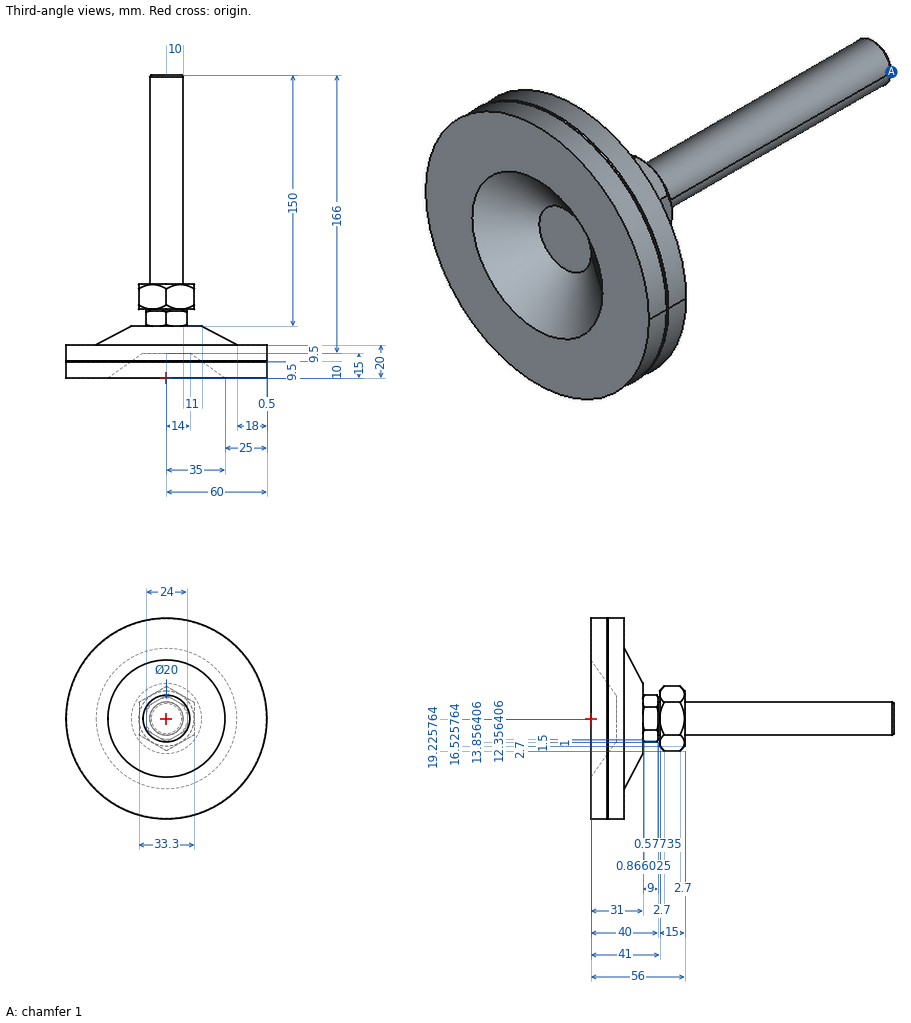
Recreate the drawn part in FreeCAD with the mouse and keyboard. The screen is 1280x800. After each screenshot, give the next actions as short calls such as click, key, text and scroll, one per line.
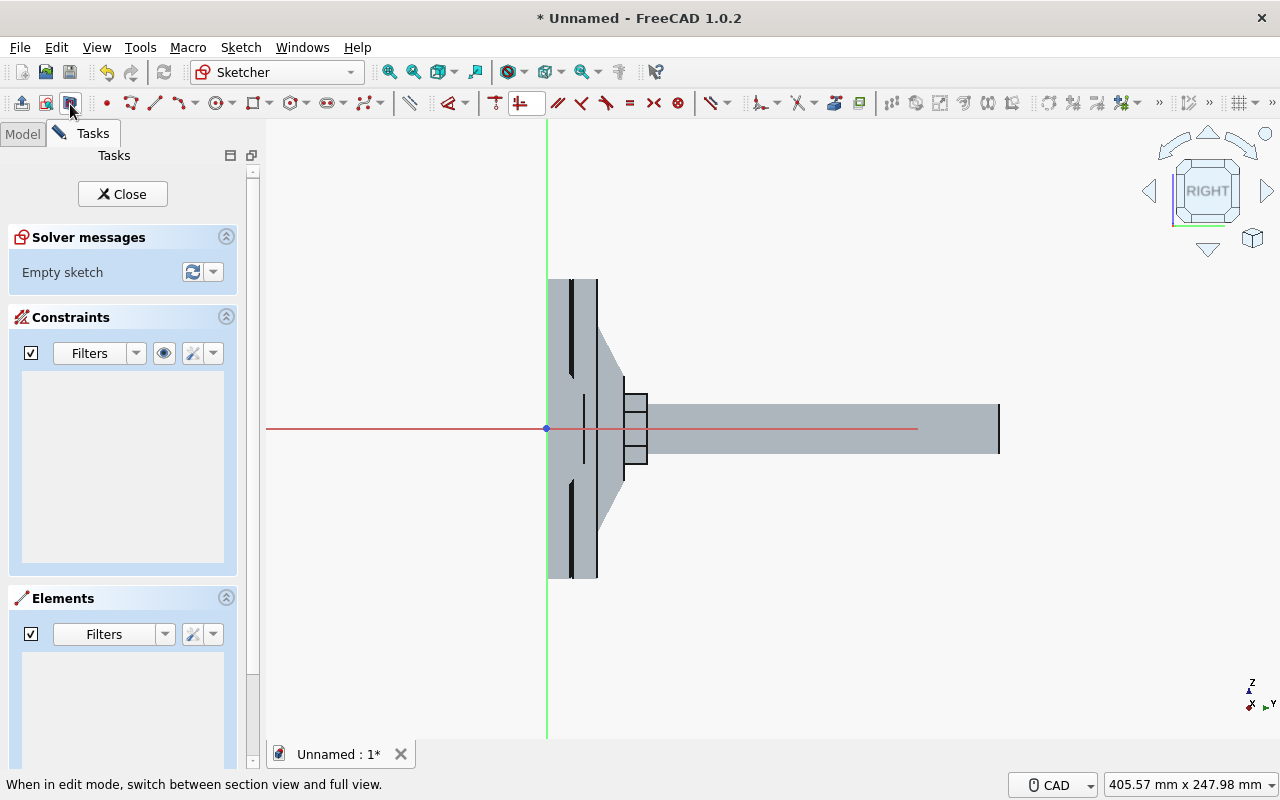
scroll(632, 463, up, 15)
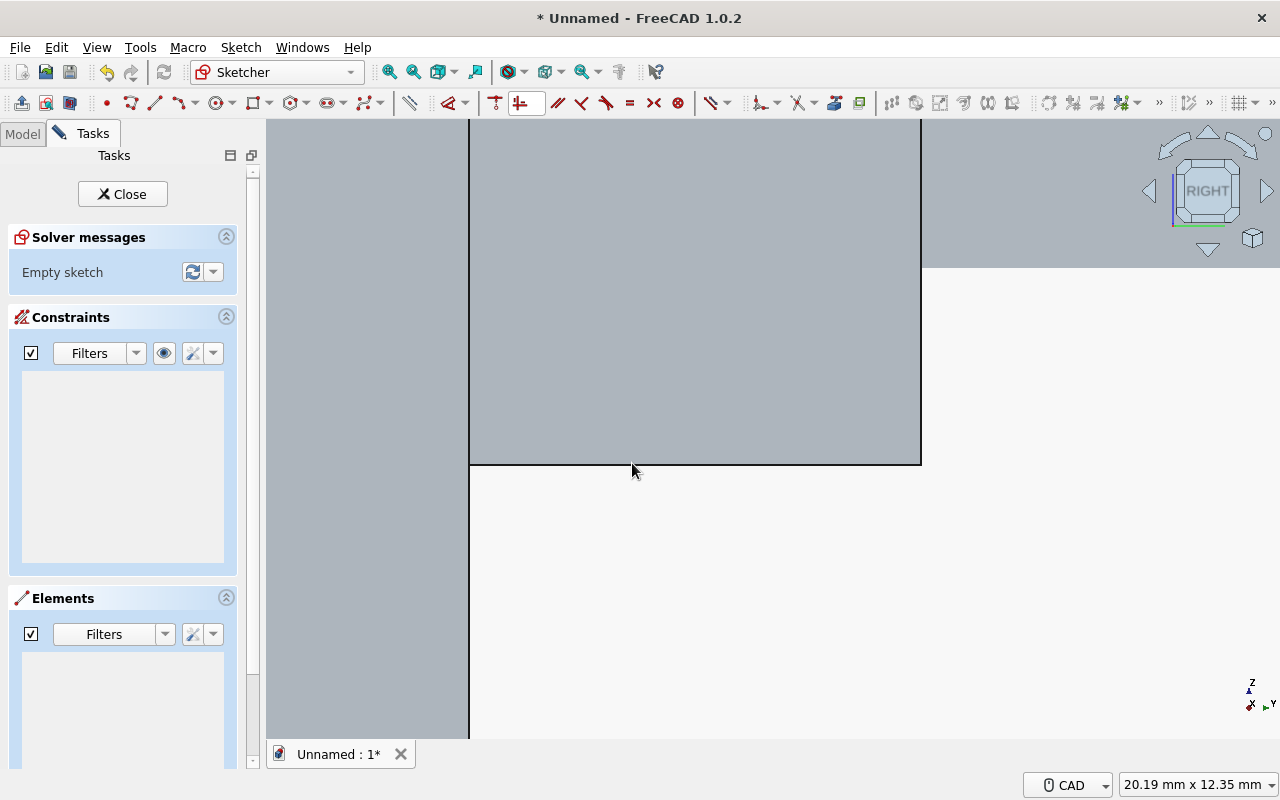
click(132, 104)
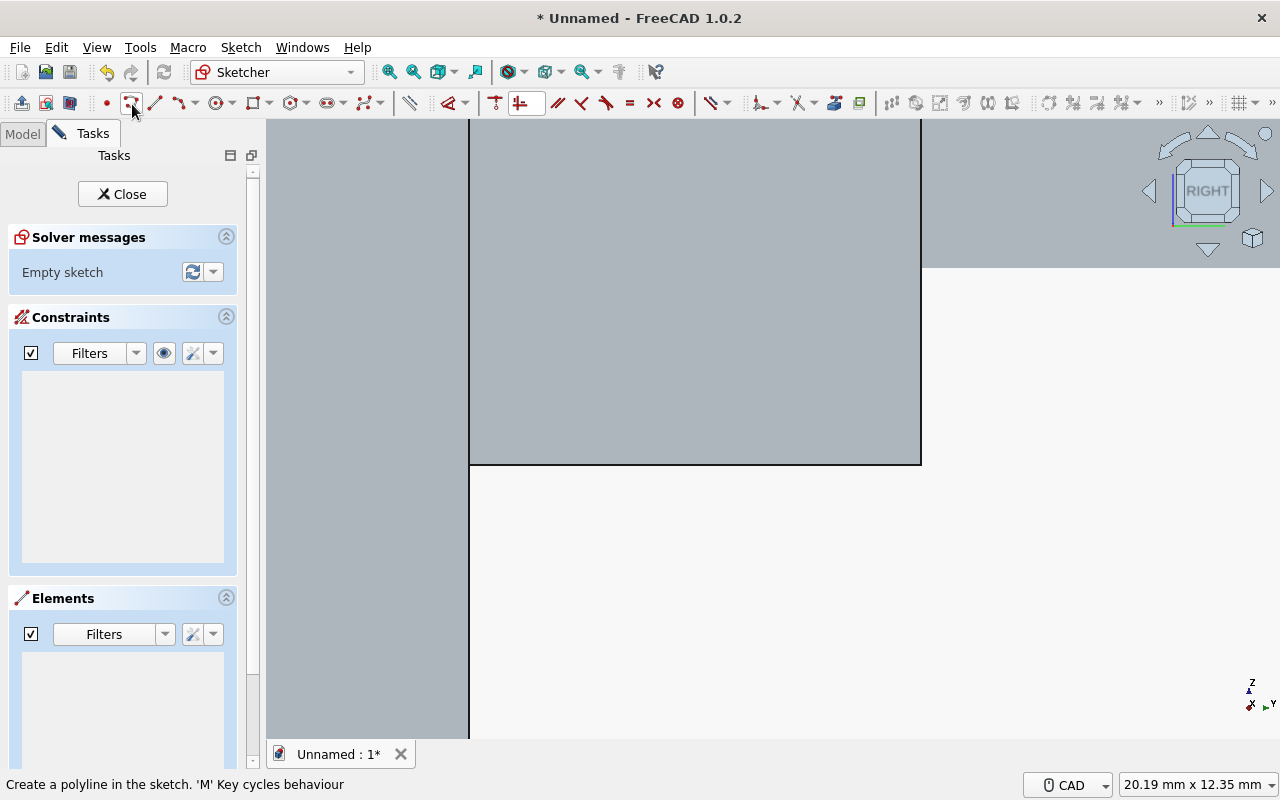
click(469, 390)
click(469, 465)
click(513, 465)
click(469, 391)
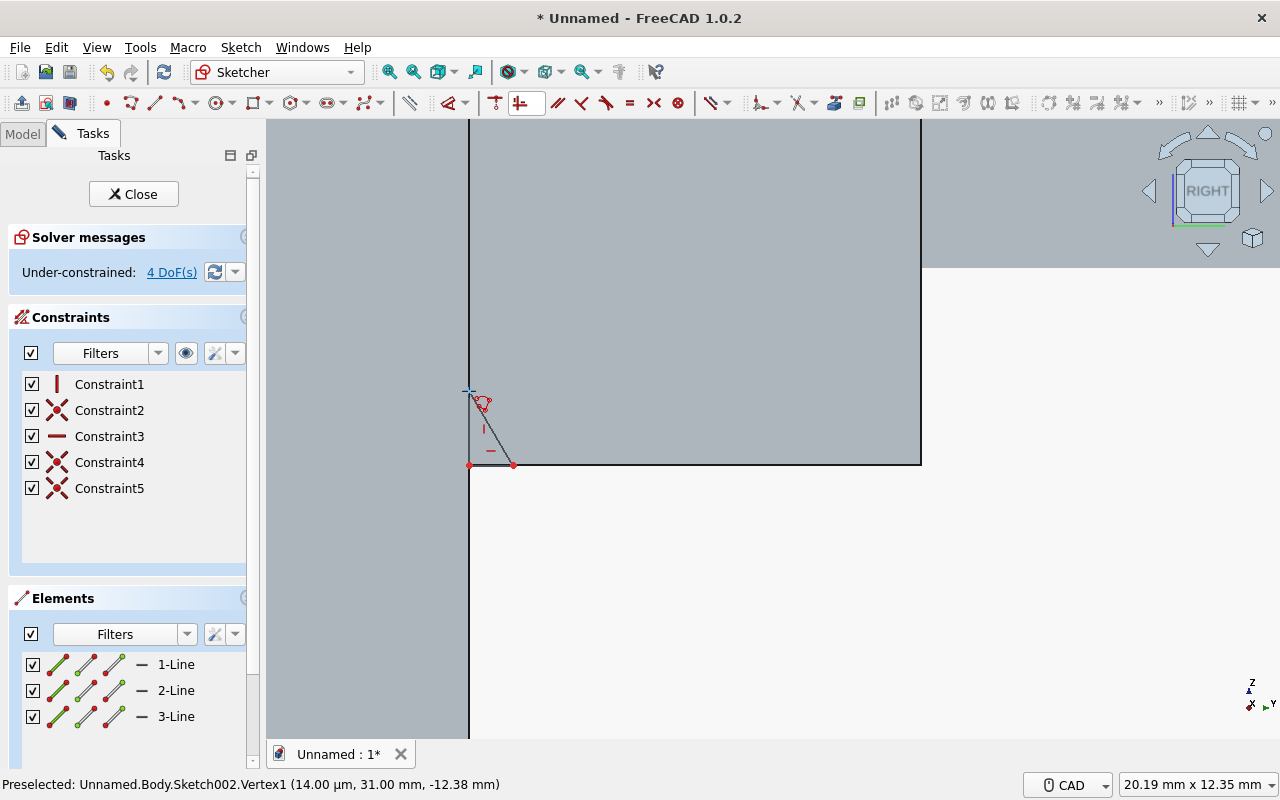
click(892, 465)
click(921, 465)
click(921, 415)
click(892, 466)
key(Escape)
key(Escape)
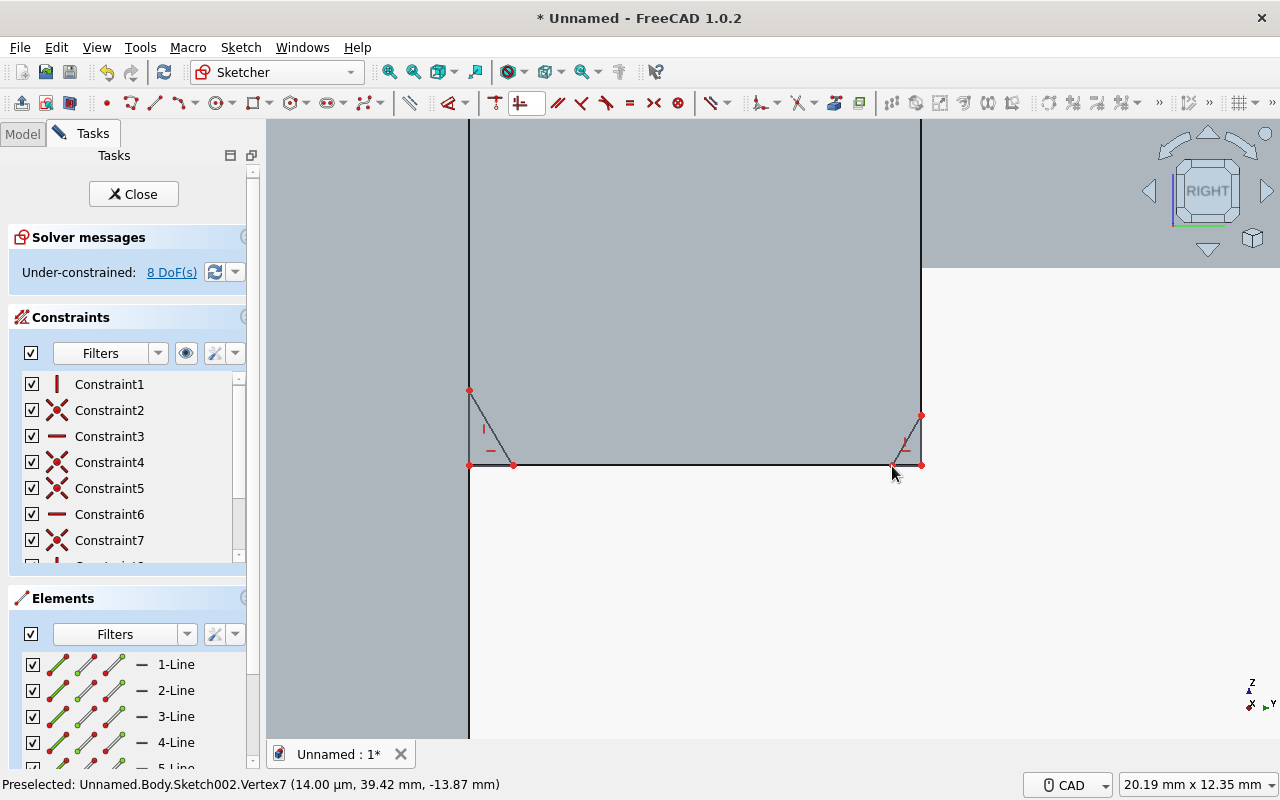
key(d)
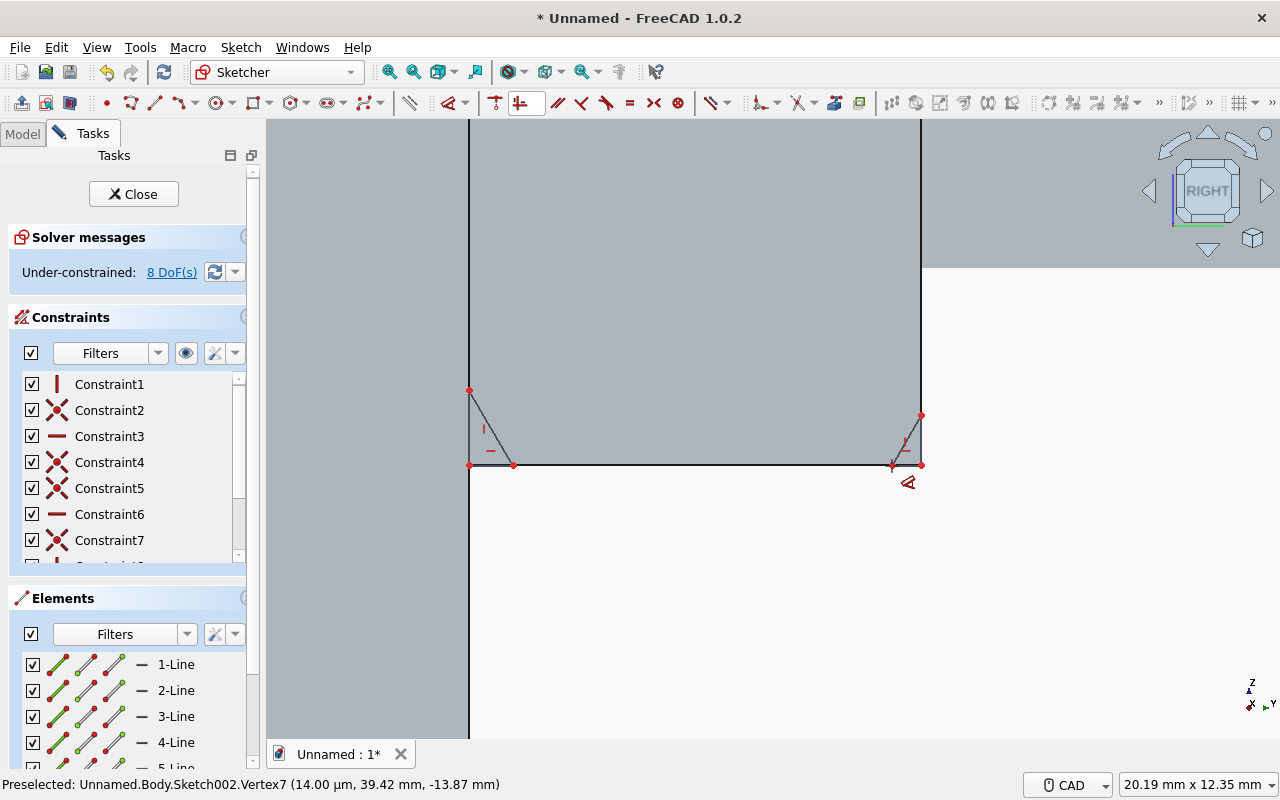
click(921, 451)
click(955, 441)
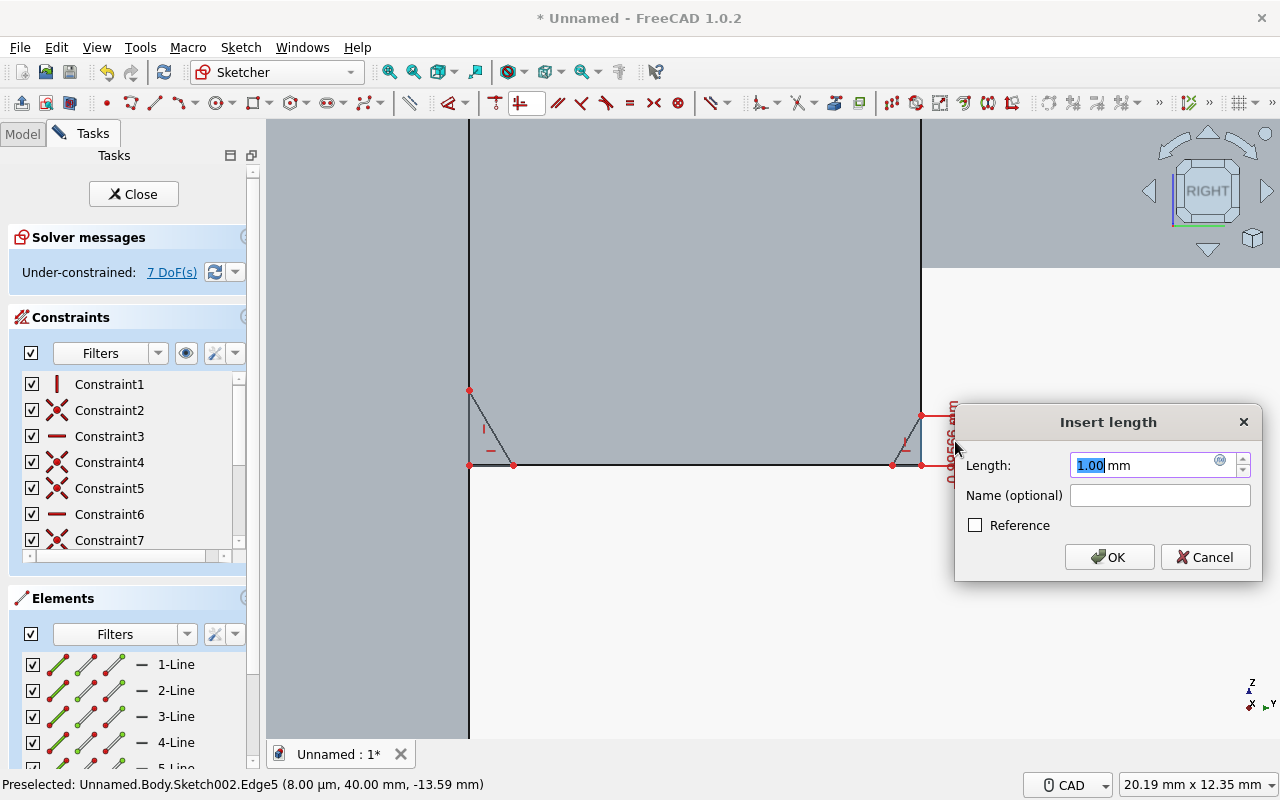
text(1)
key(Return)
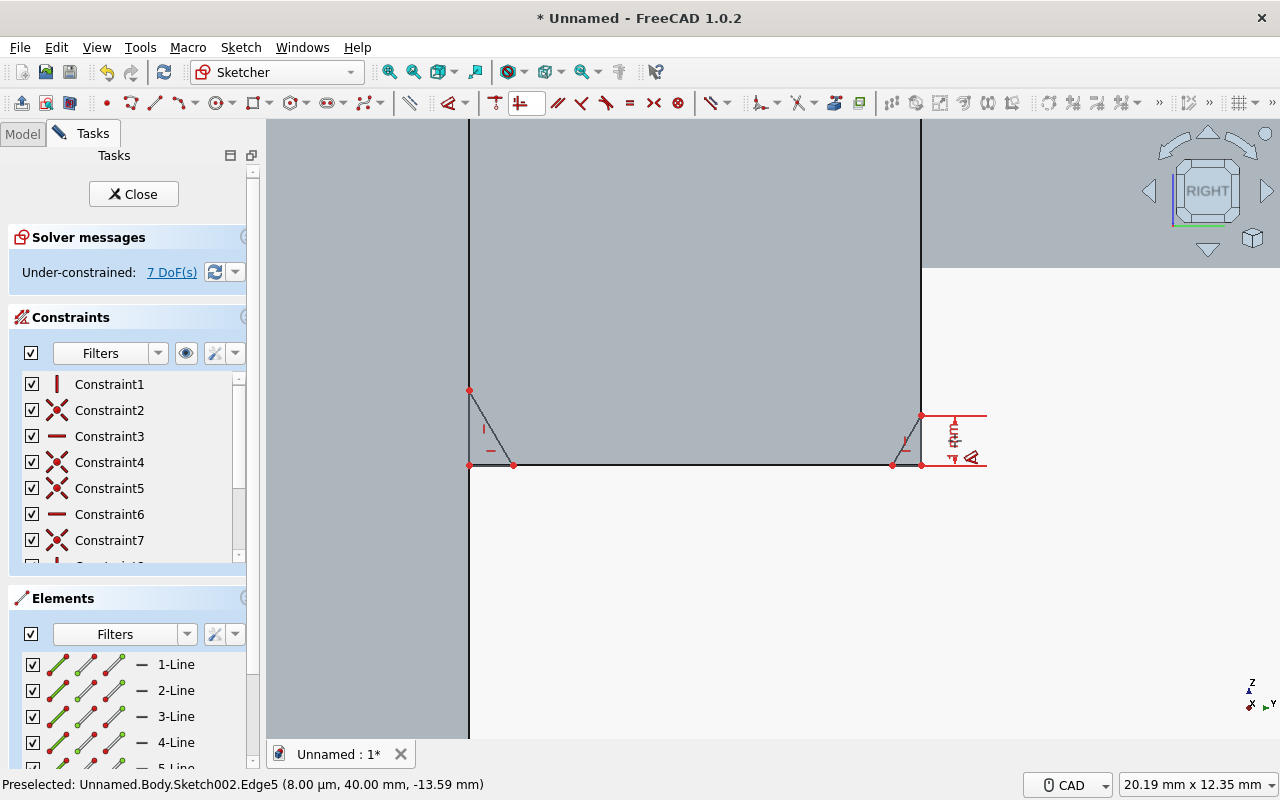
click(469, 413)
click(435, 429)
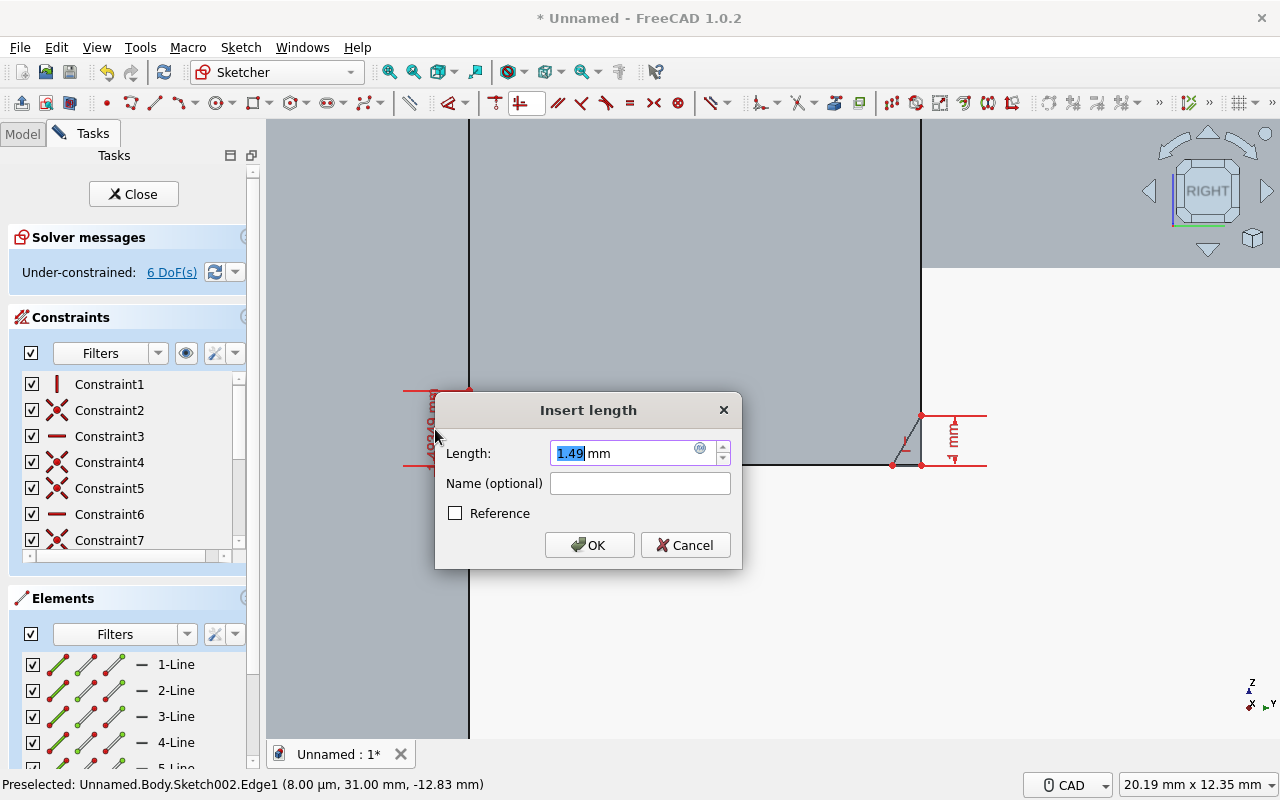
text(1.5)
key(Return)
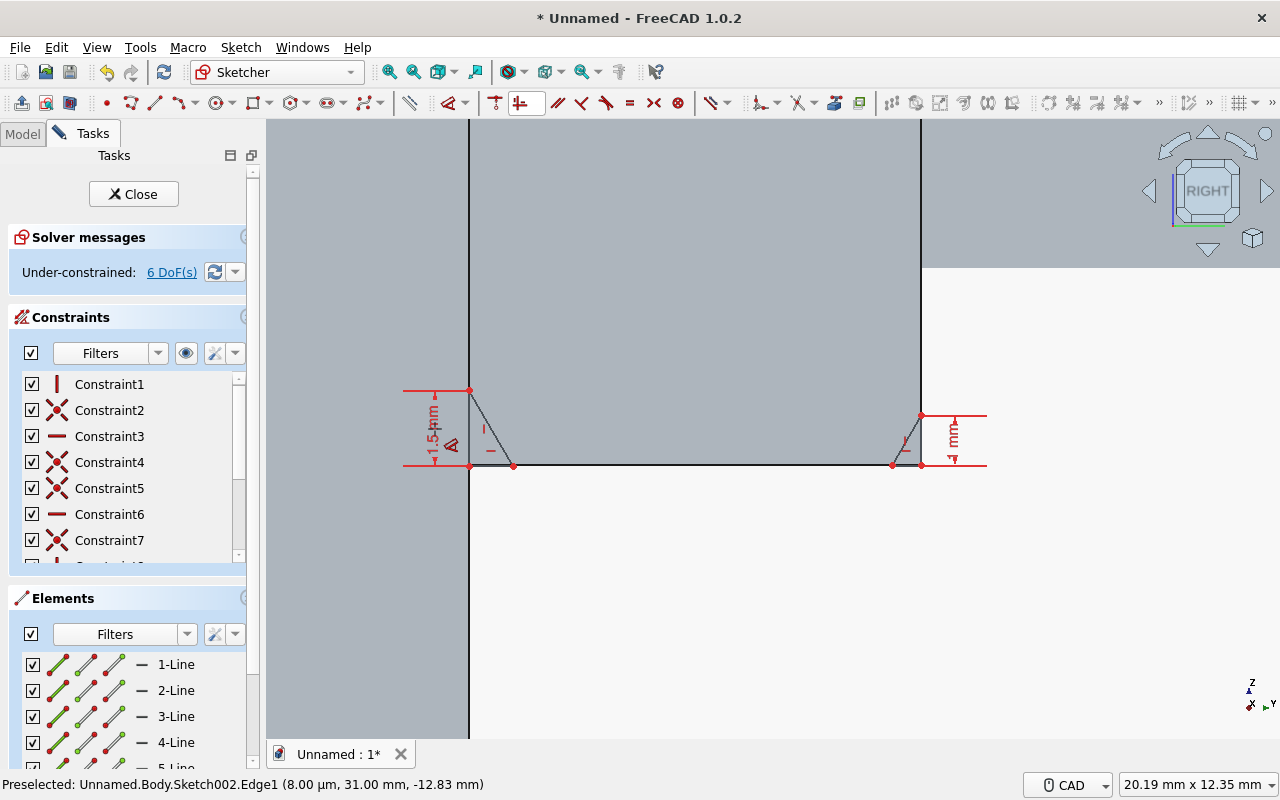
click(469, 391)
click(341, 425)